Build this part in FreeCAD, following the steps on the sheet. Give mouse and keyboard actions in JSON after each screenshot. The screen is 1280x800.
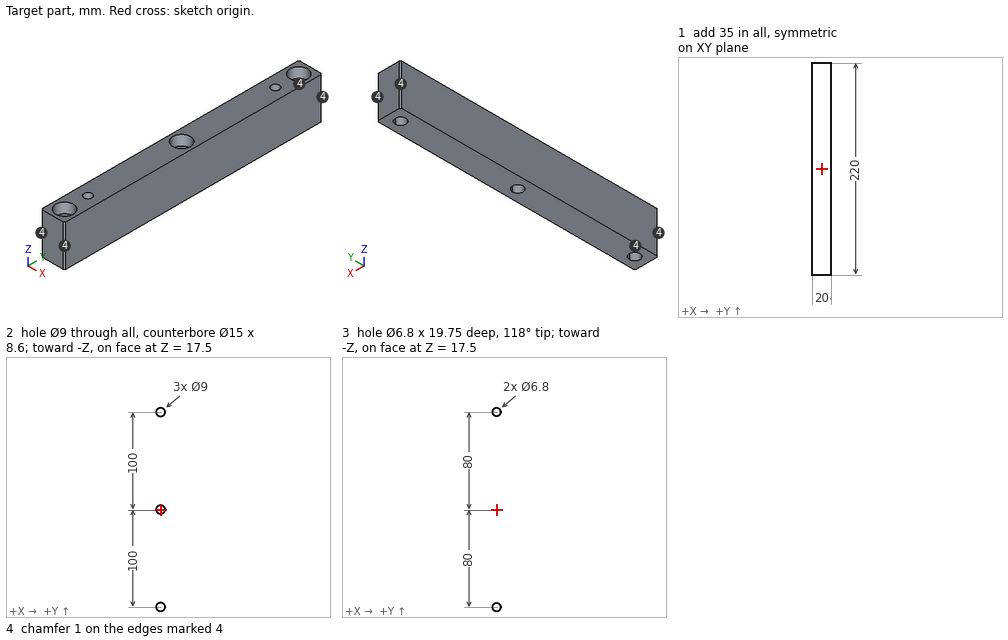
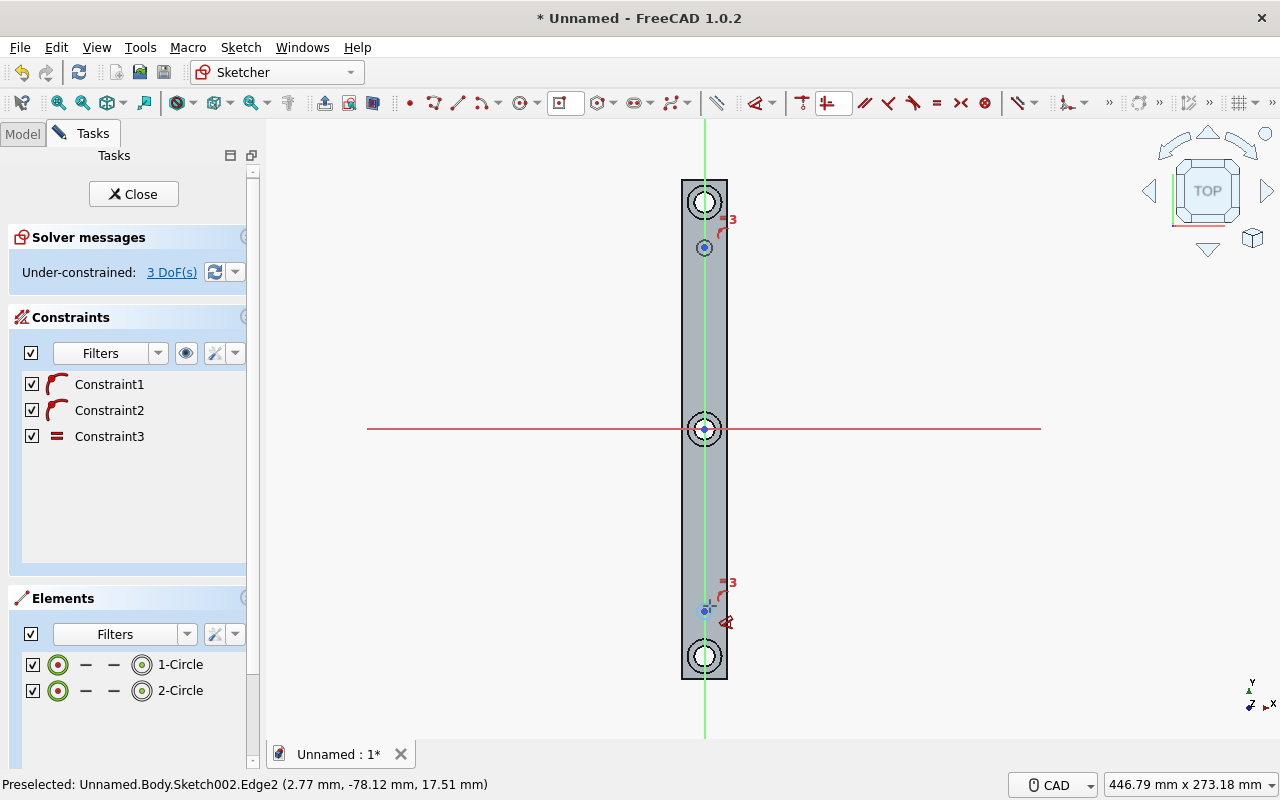
{"action": "scroll", "coordinate": [710, 243], "scroll_direction": "up", "scroll_amount": 5}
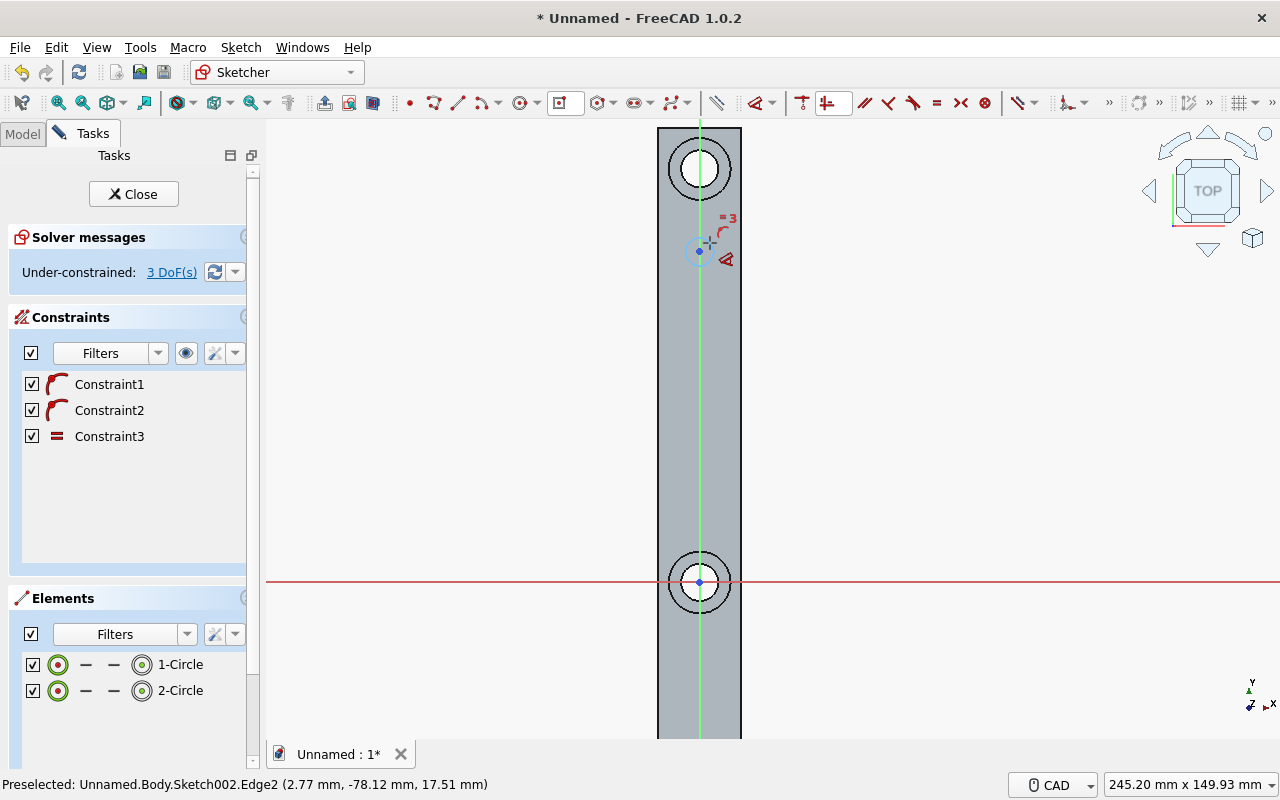
{"action": "left_click", "coordinate": [709, 242]}
{"action": "left_click", "coordinate": [732, 220]}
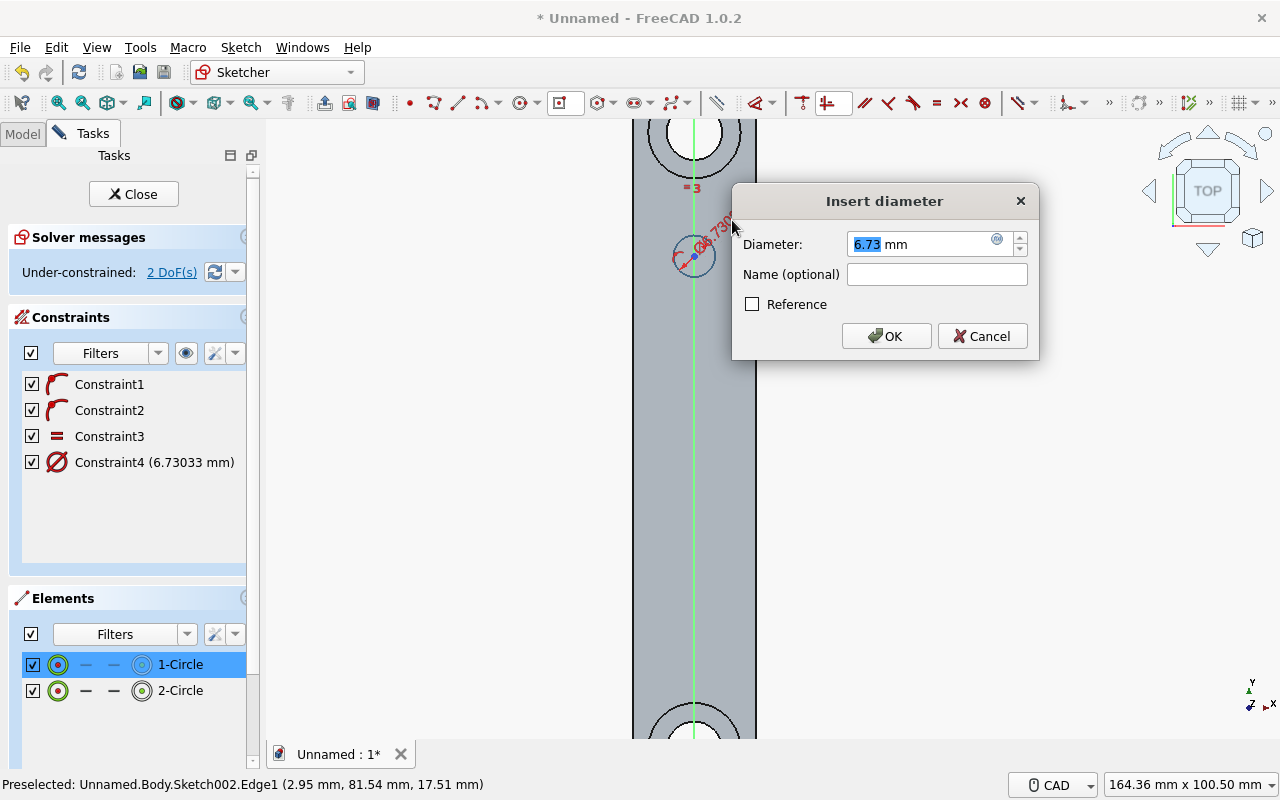
{"action": "type", "text": "6.8"}
{"action": "key", "text": "Return"}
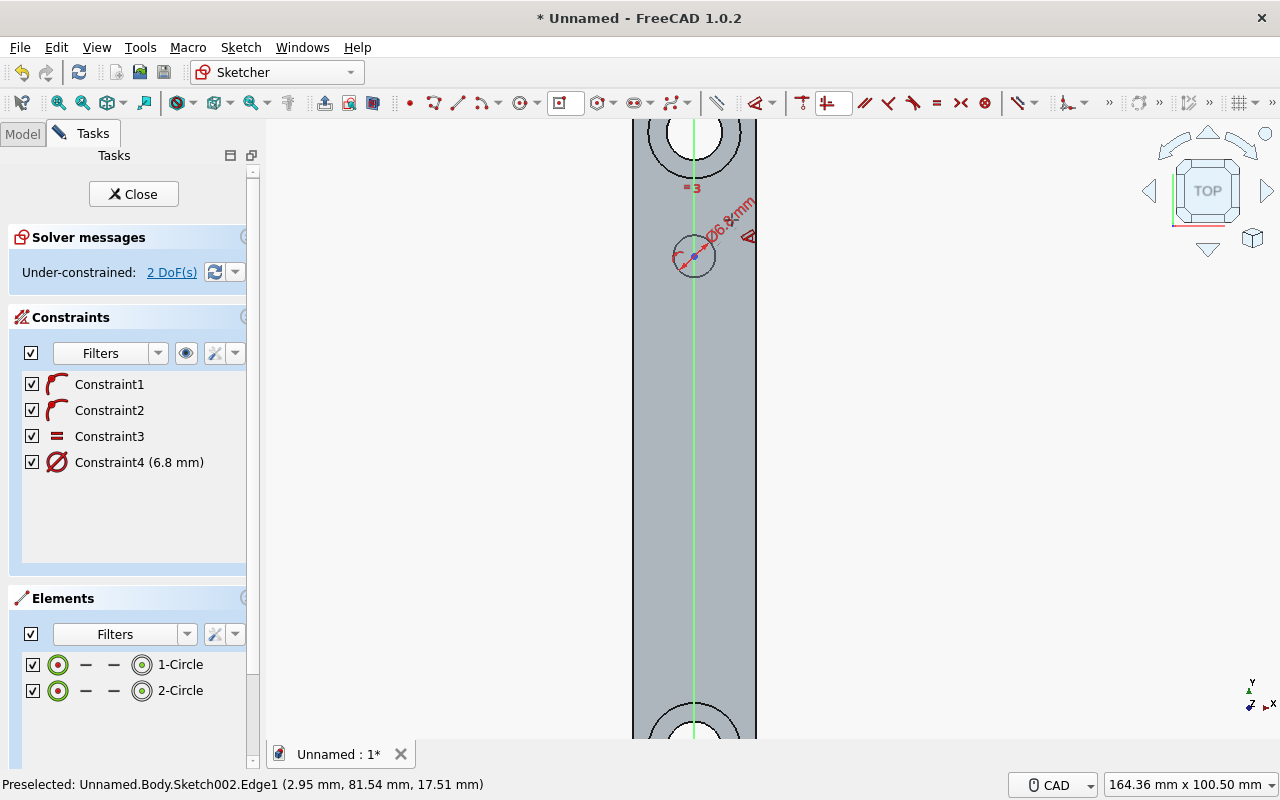
{"action": "left_click", "coordinate": [694, 256]}
{"action": "left_click", "coordinate": [728, 484]}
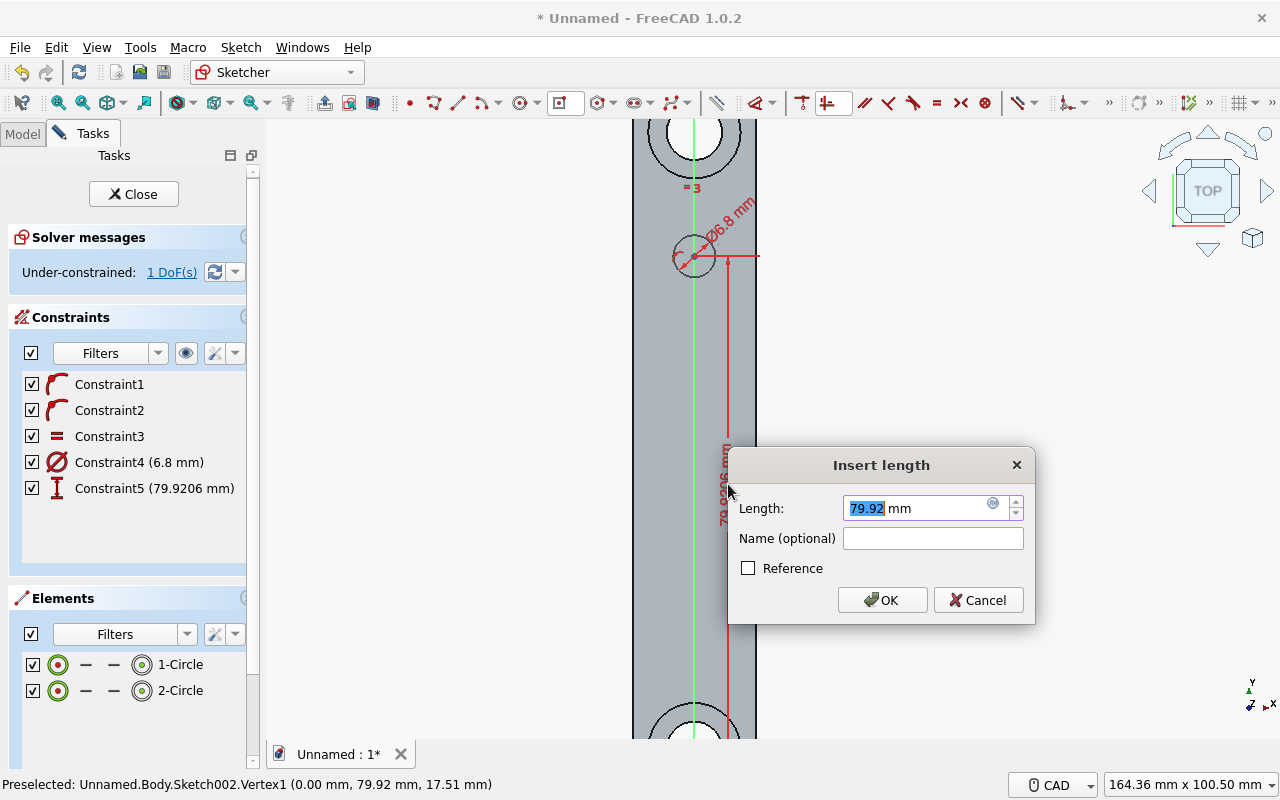
{"action": "type", "text": "80"}
{"action": "key", "text": "Return"}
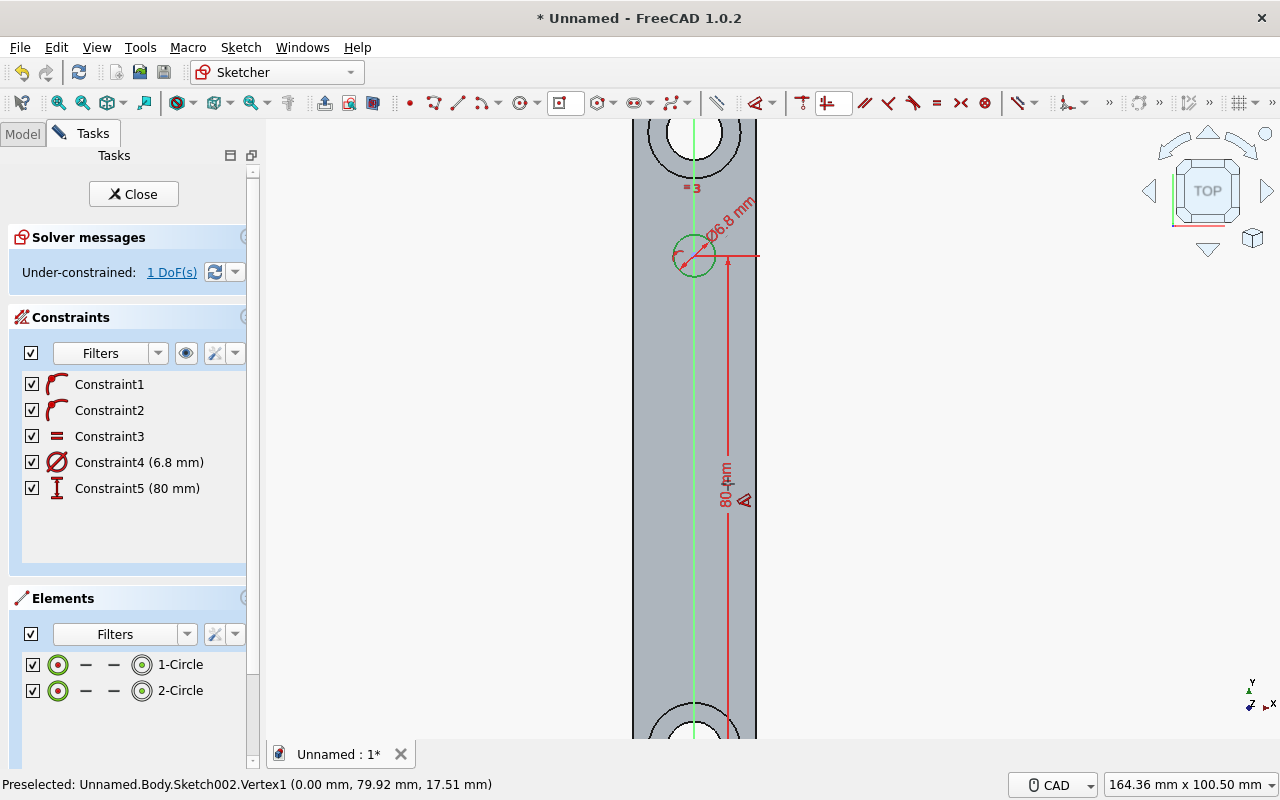
{"action": "scroll", "coordinate": [710, 243], "scroll_direction": "down", "scroll_amount": 5}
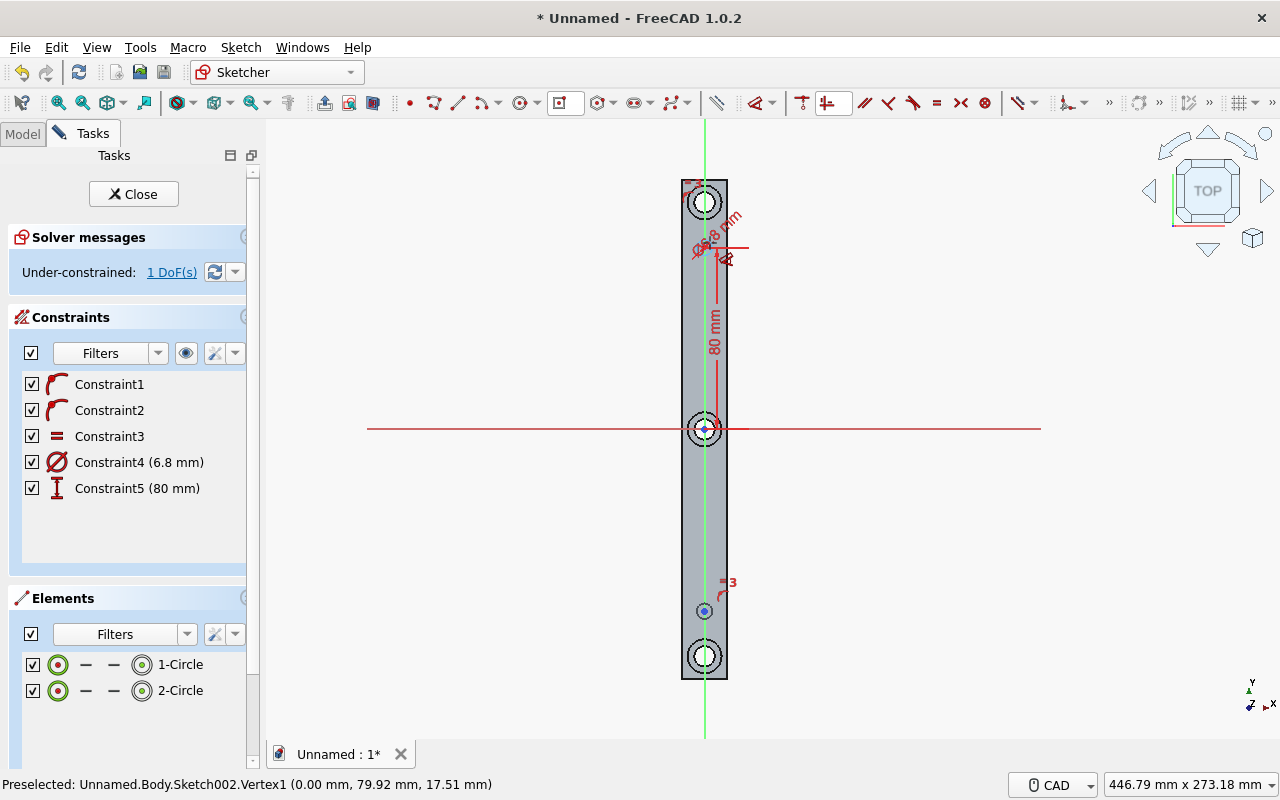
{"action": "left_click", "coordinate": [705, 611]}
{"action": "left_click", "coordinate": [739, 520]}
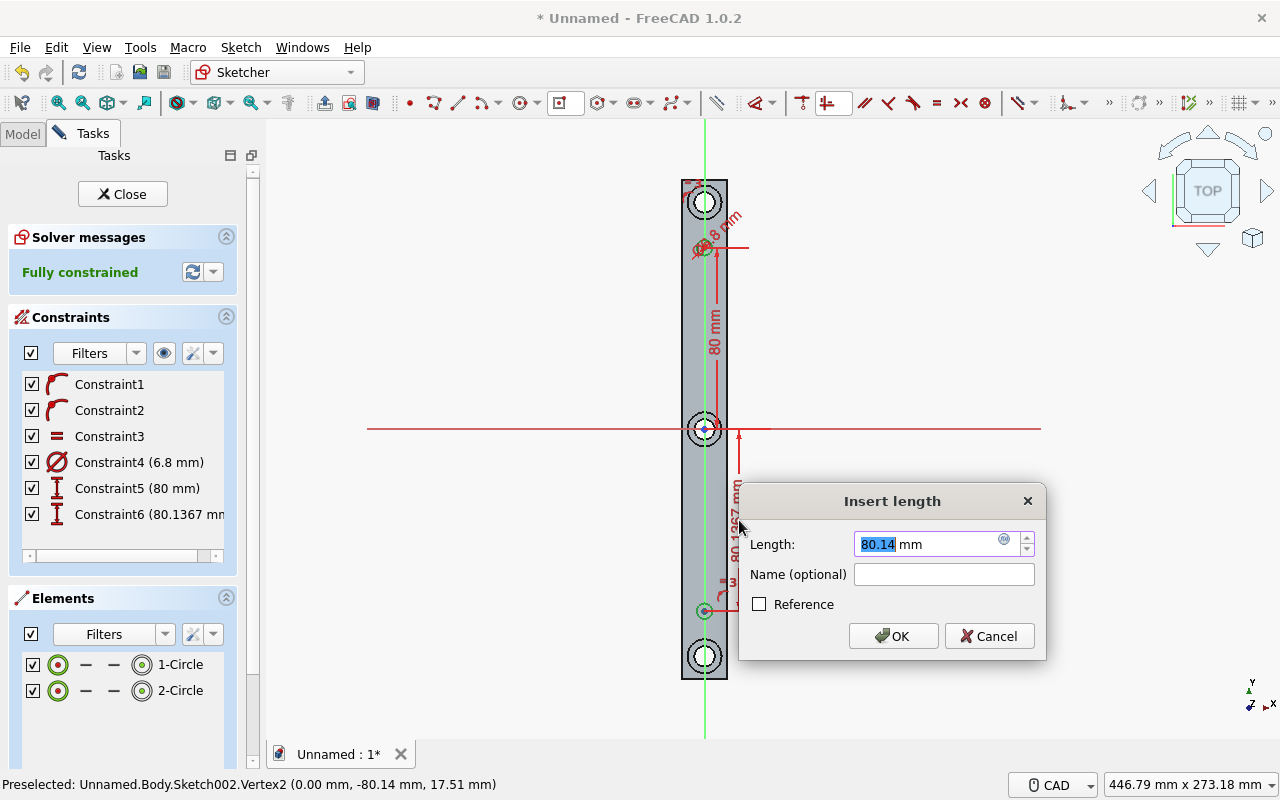
{"action": "type", "text": "80"}
{"action": "key", "text": "Return"}
{"action": "key", "text": "Escape"}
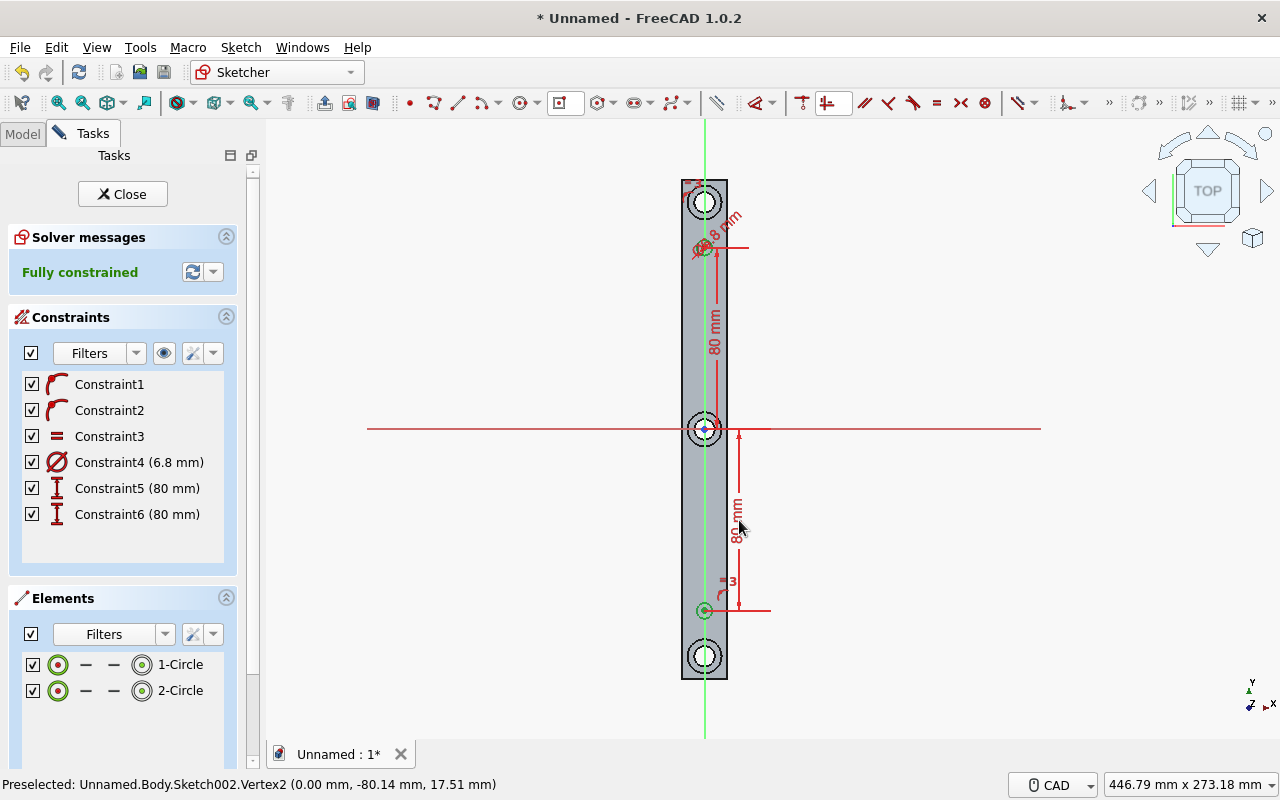
{"action": "left_click", "coordinate": [123, 194]}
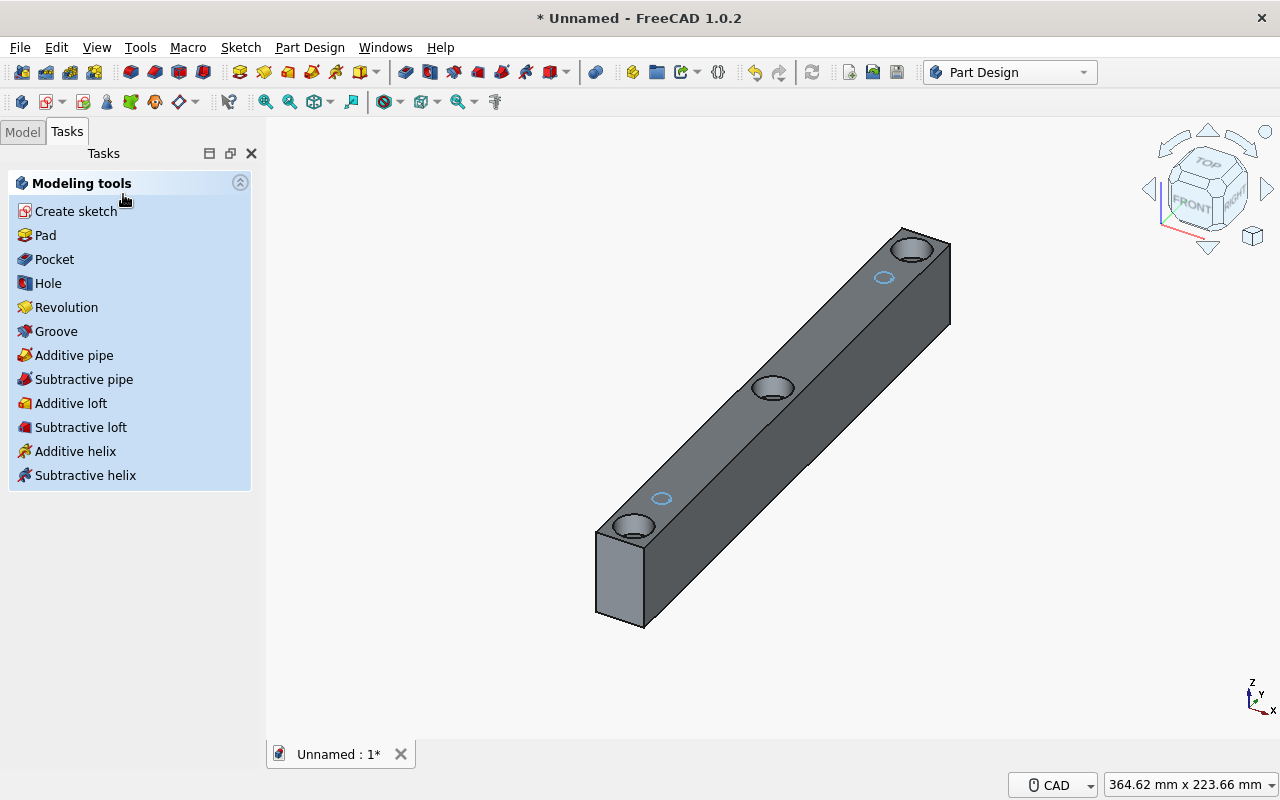
{"action": "left_click", "coordinate": [430, 72]}